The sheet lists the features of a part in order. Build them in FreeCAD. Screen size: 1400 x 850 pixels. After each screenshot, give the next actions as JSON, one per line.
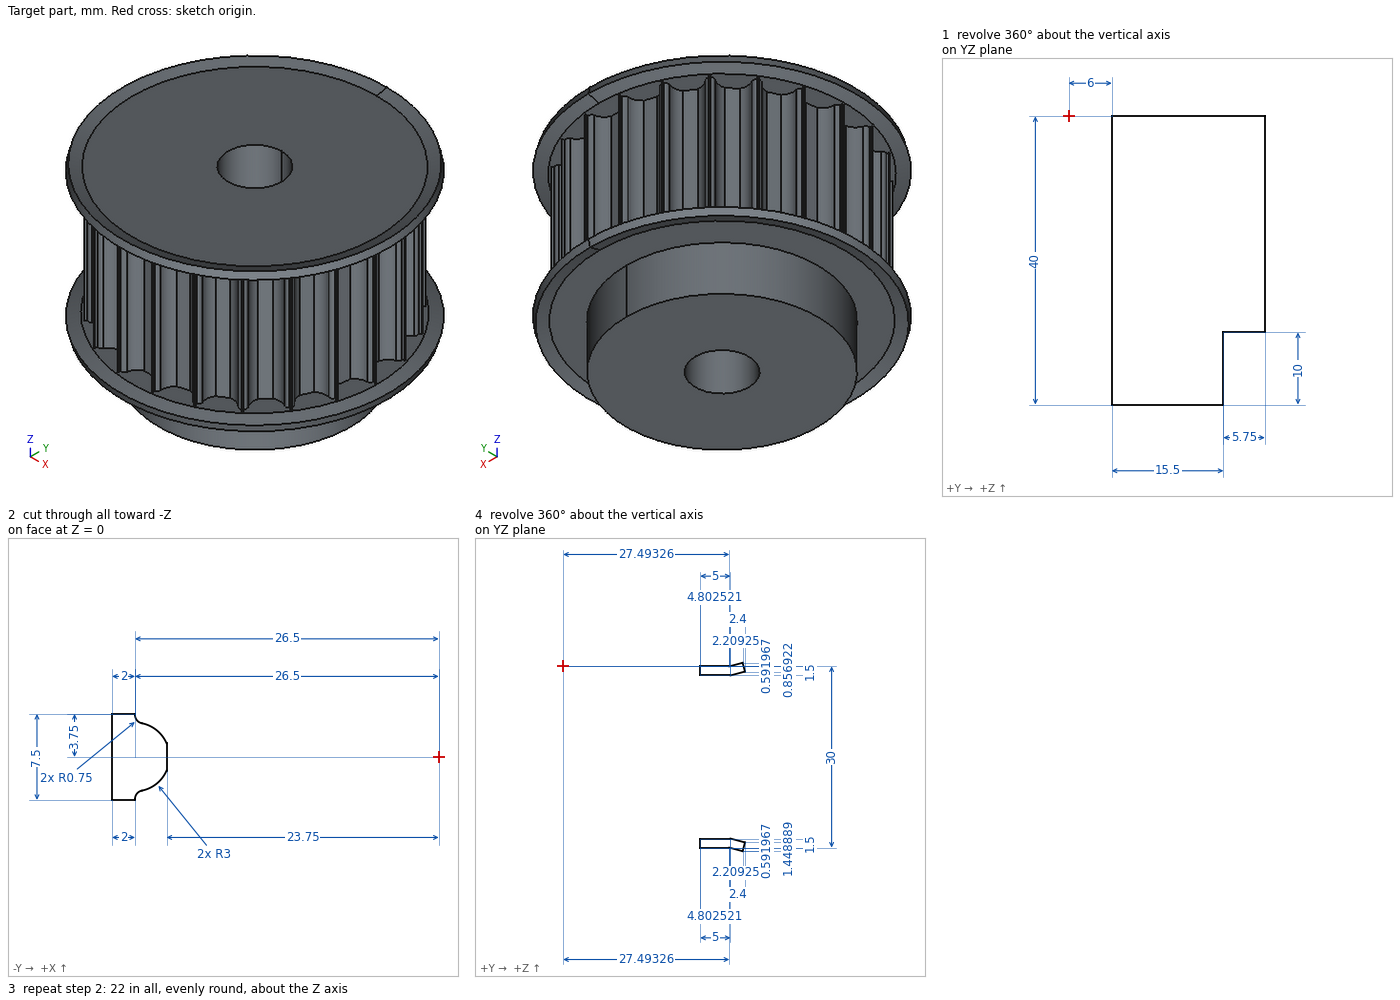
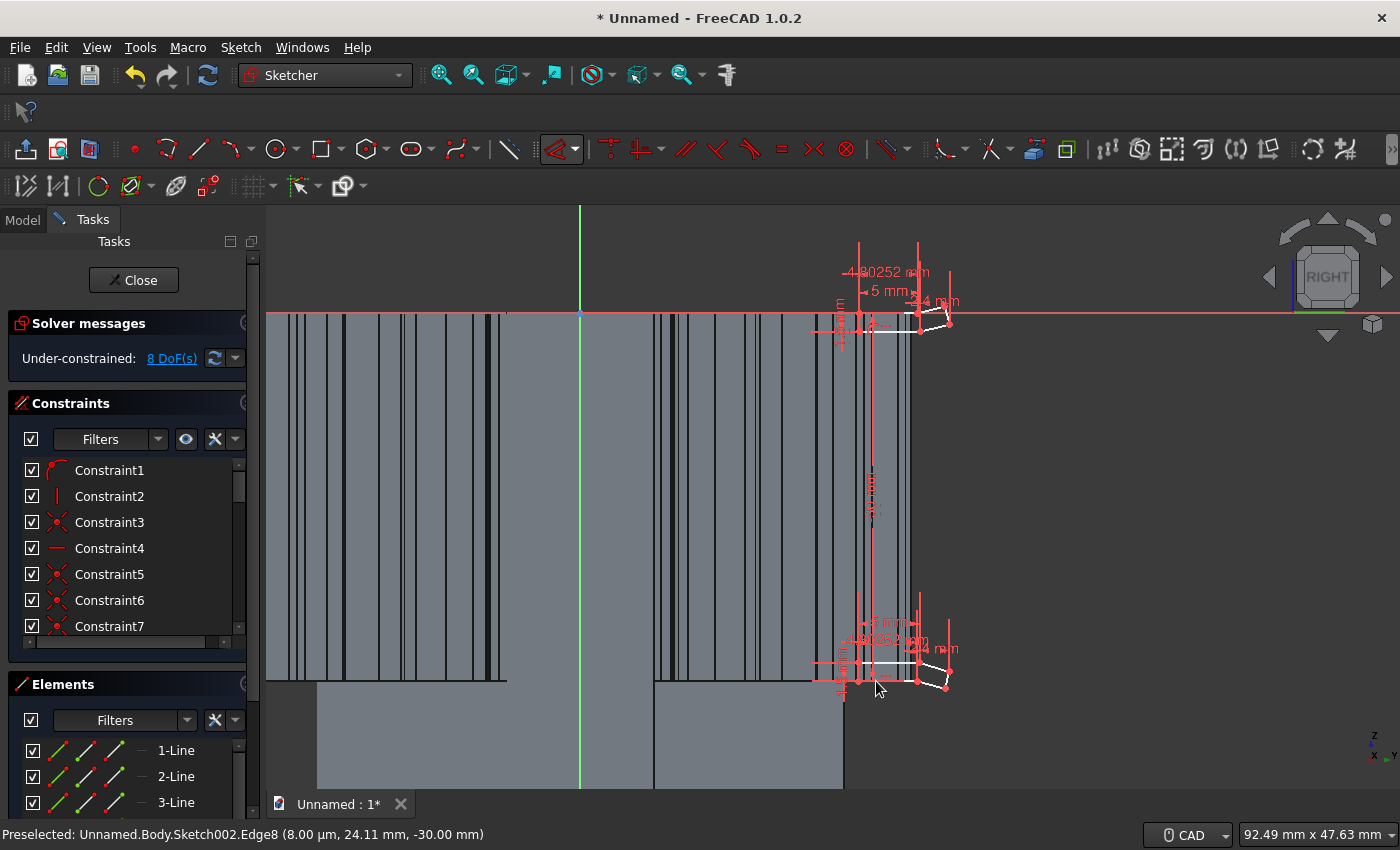
{"action": "scroll", "coordinate": [929, 311], "scroll_direction": "up", "scroll_amount": 2}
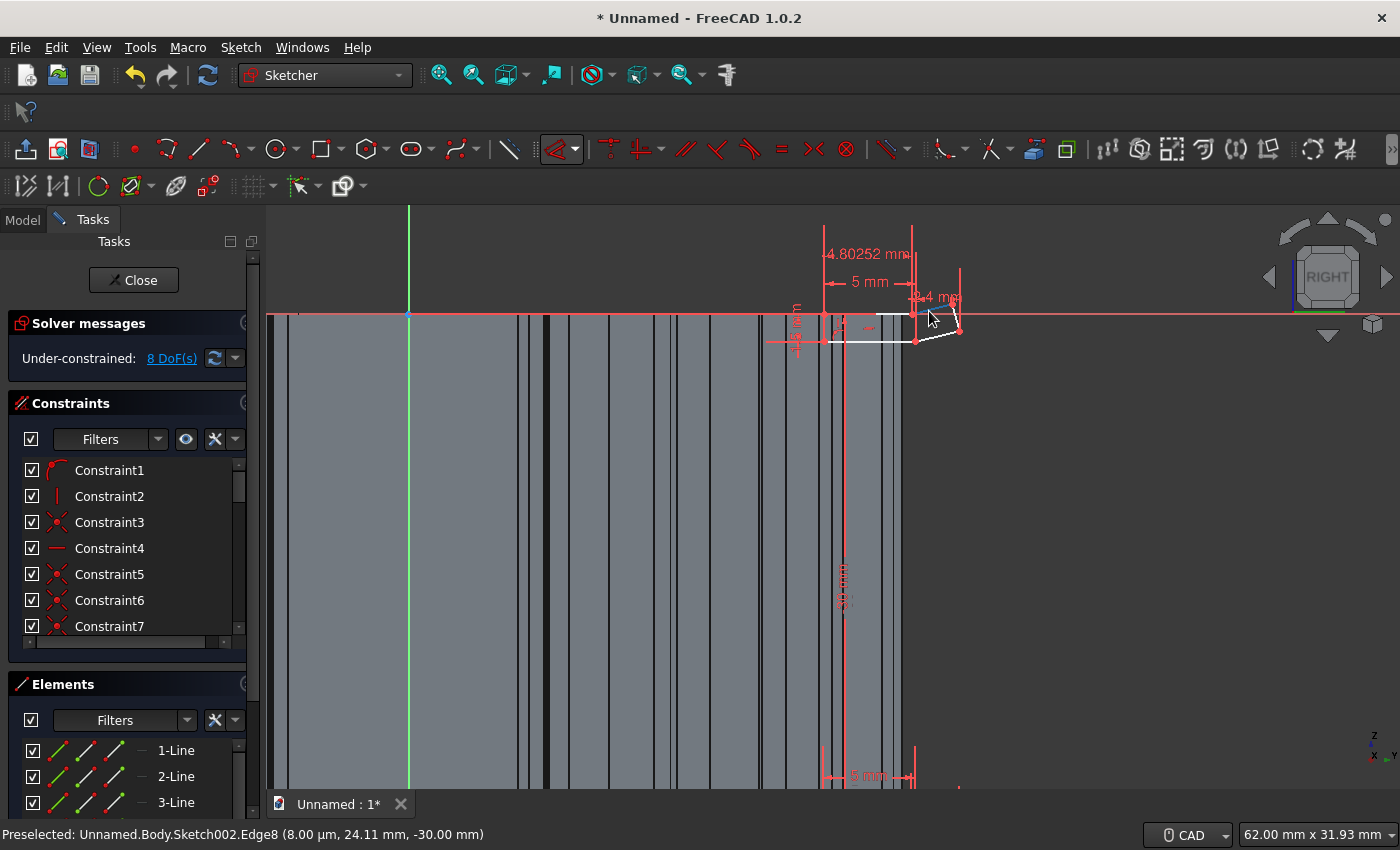
{"action": "left_click", "coordinate": [928, 310]}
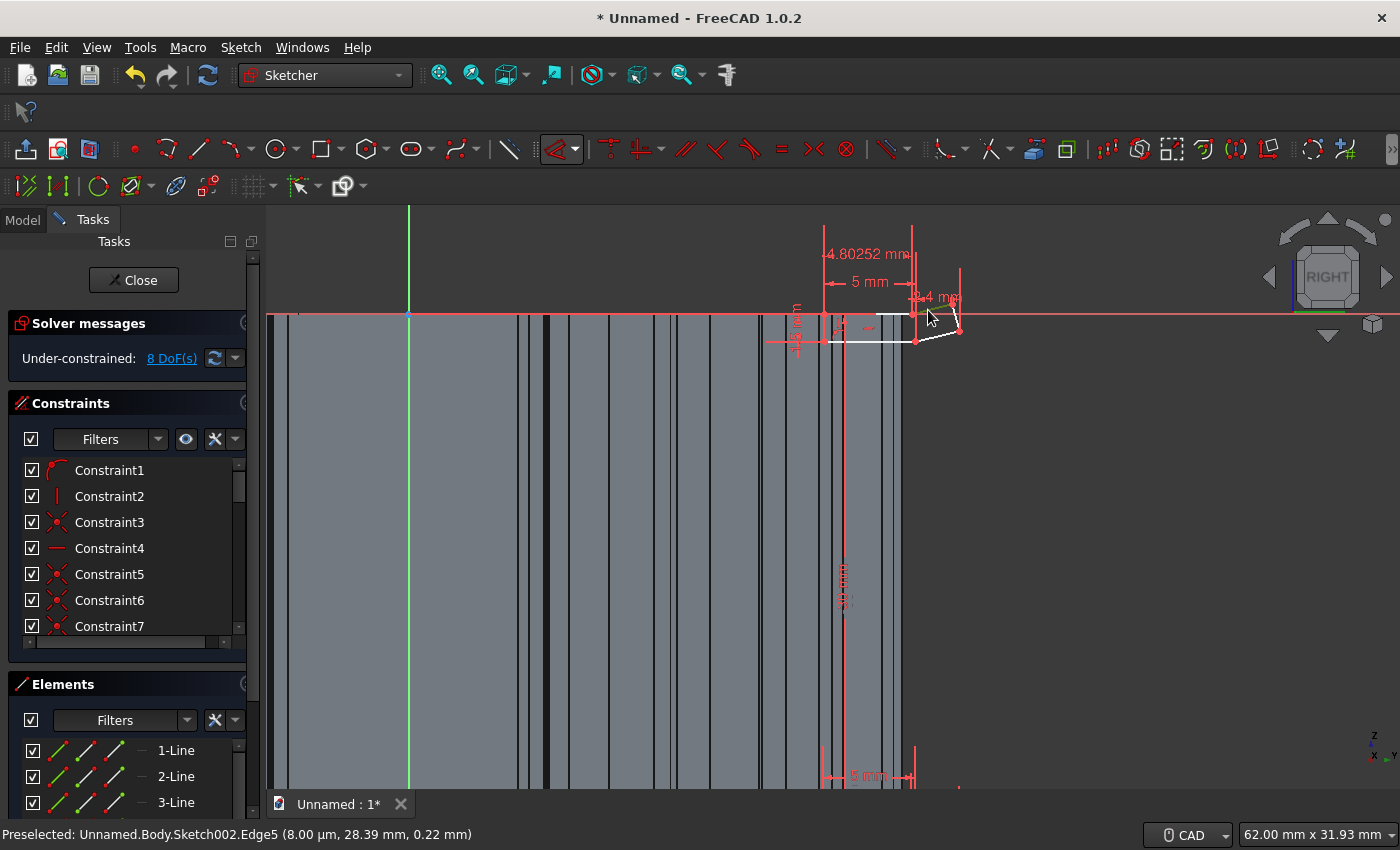
{"action": "key", "text": "l"}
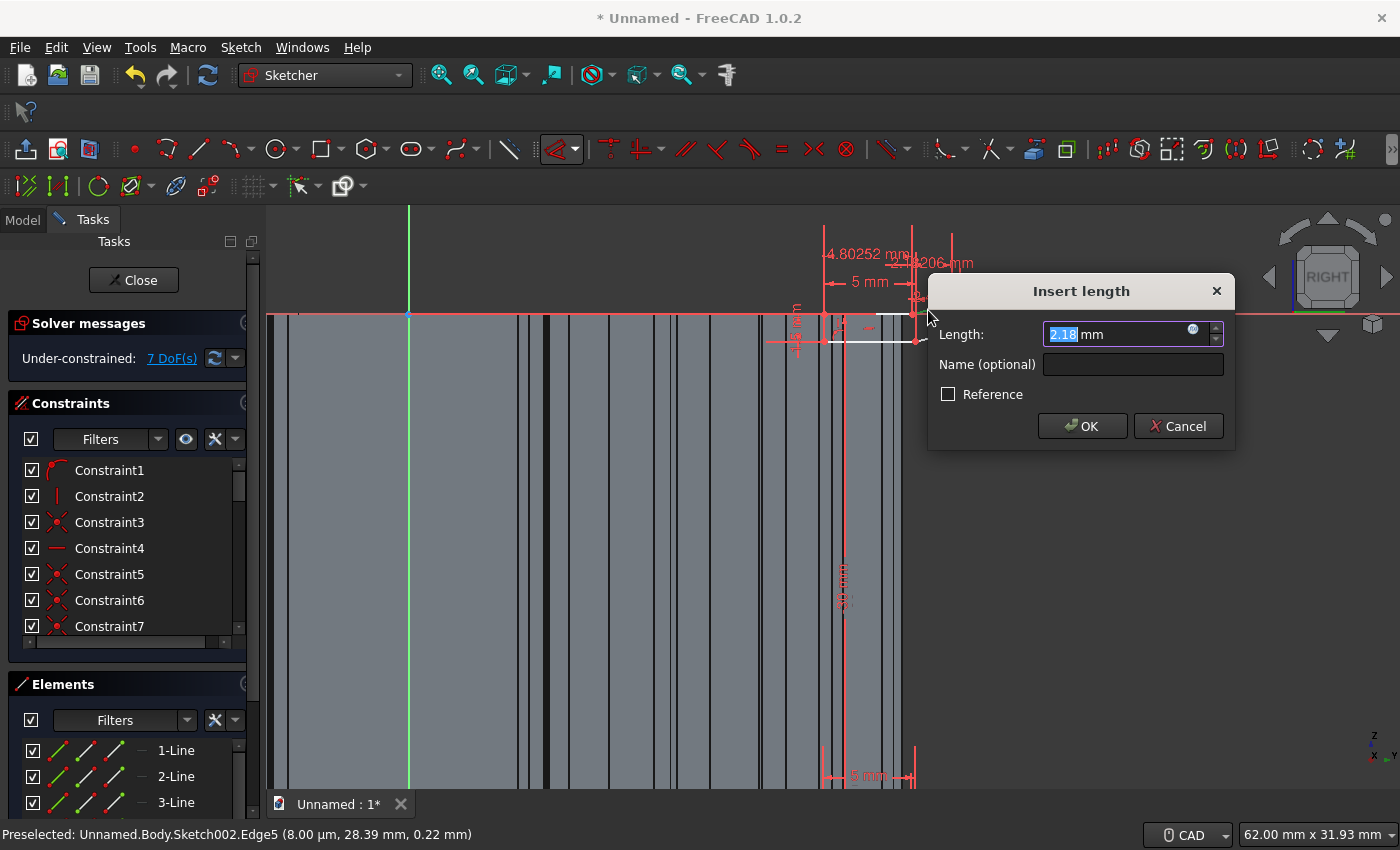
{"action": "type", "text": "2.20925"}
{"action": "key", "text": "Return"}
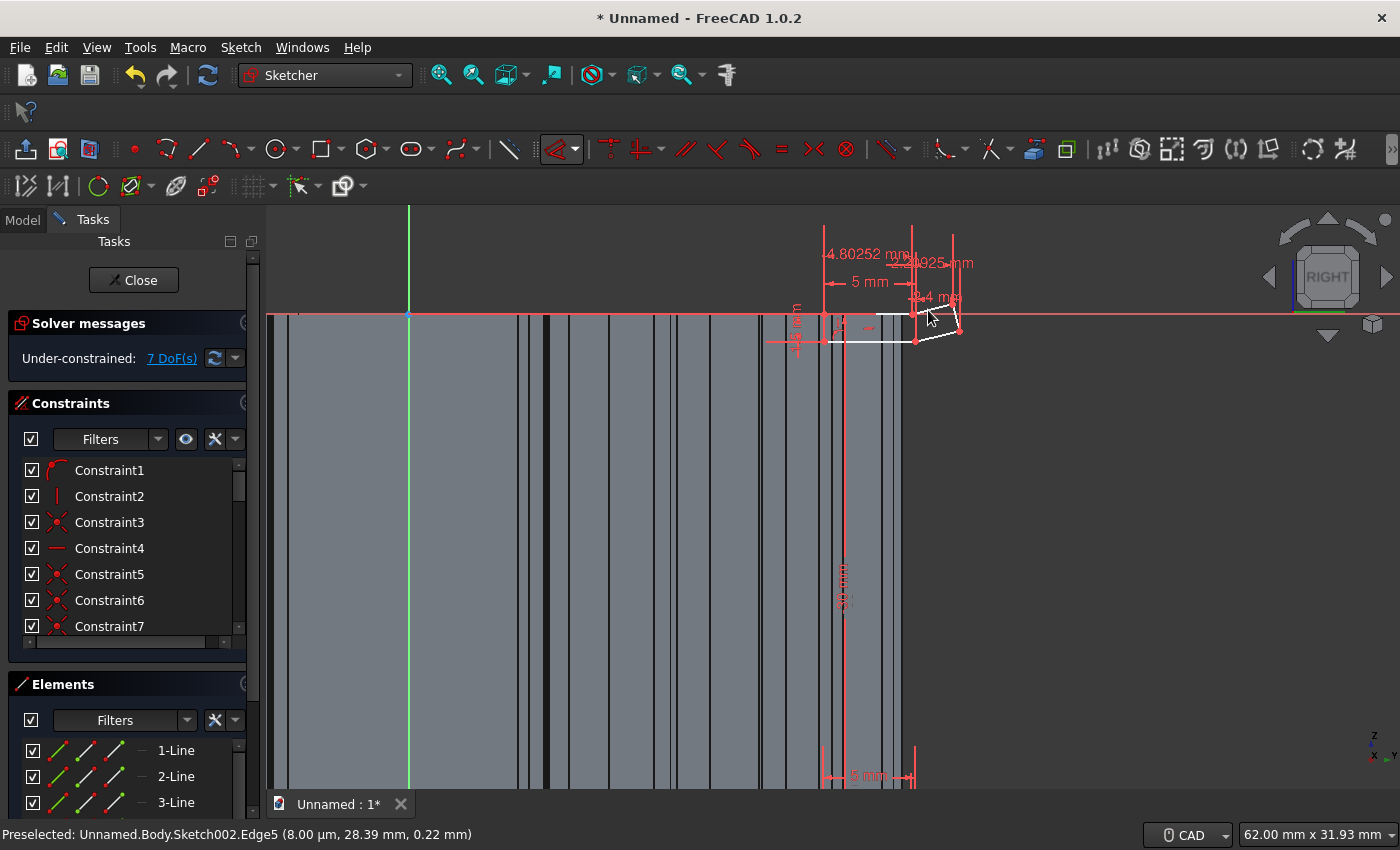
{"action": "scroll", "coordinate": [929, 310], "scroll_direction": "down", "scroll_amount": 2}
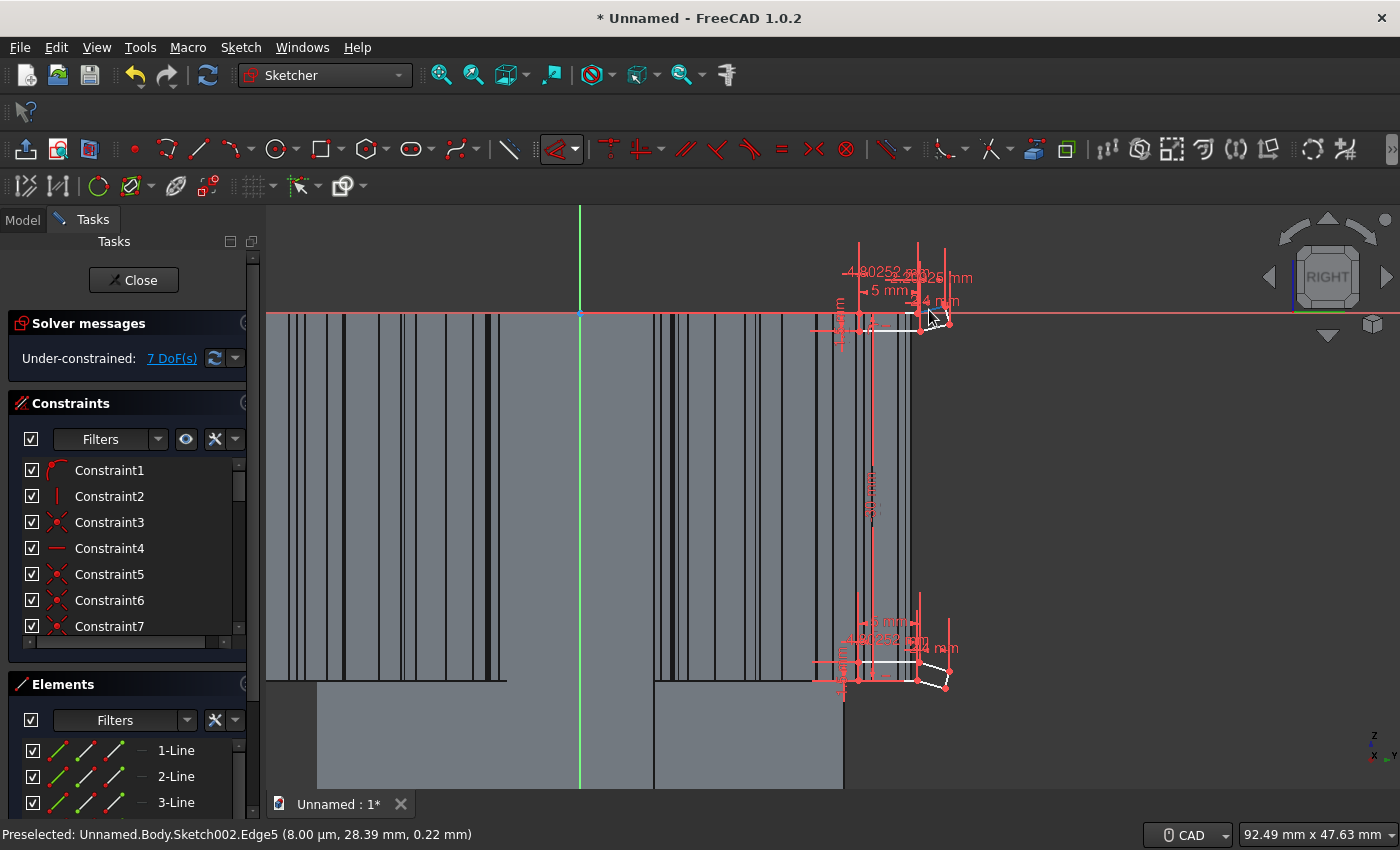
{"action": "scroll", "coordinate": [926, 683], "scroll_direction": "up", "scroll_amount": 3}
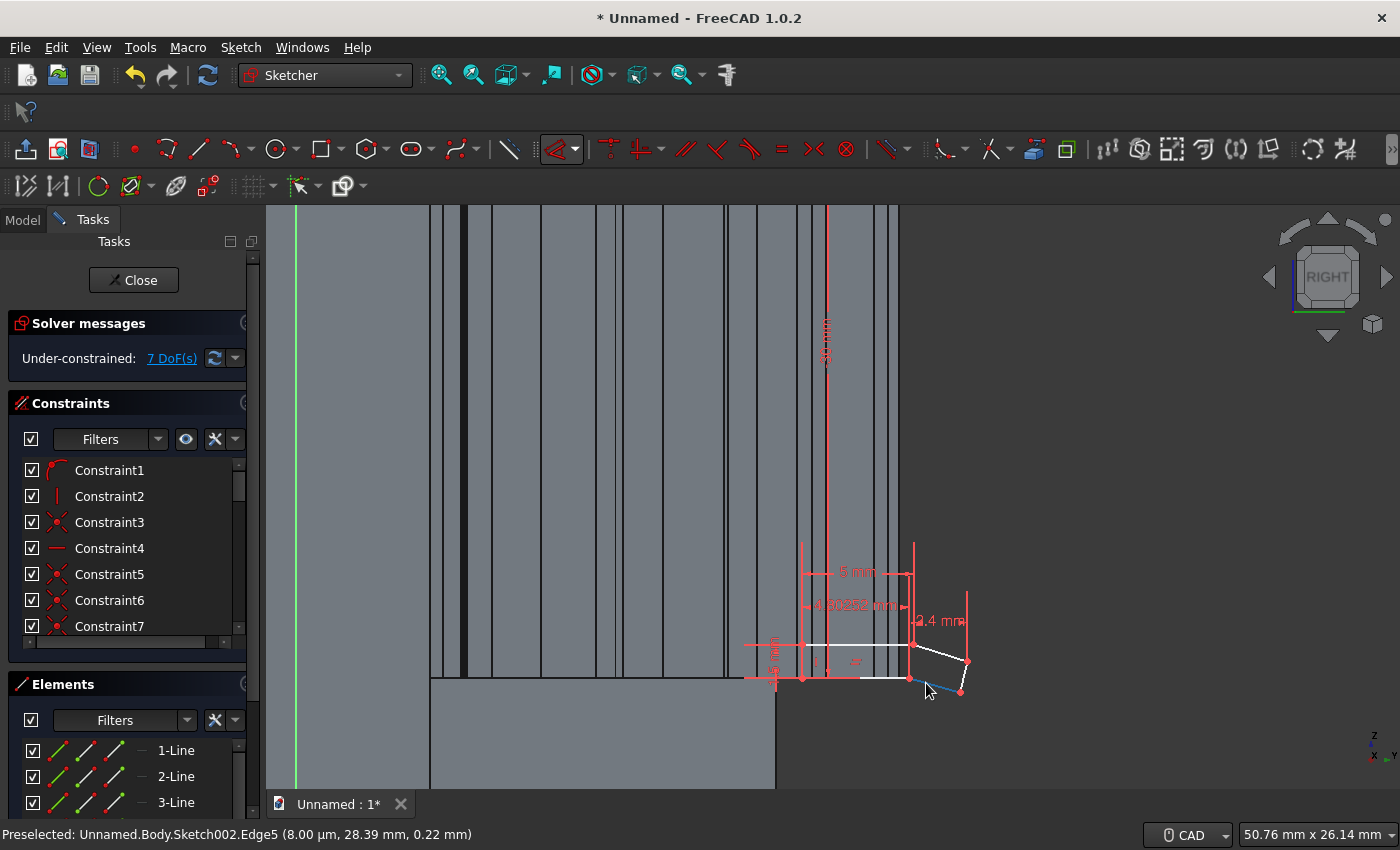
{"action": "left_click", "coordinate": [925, 683]}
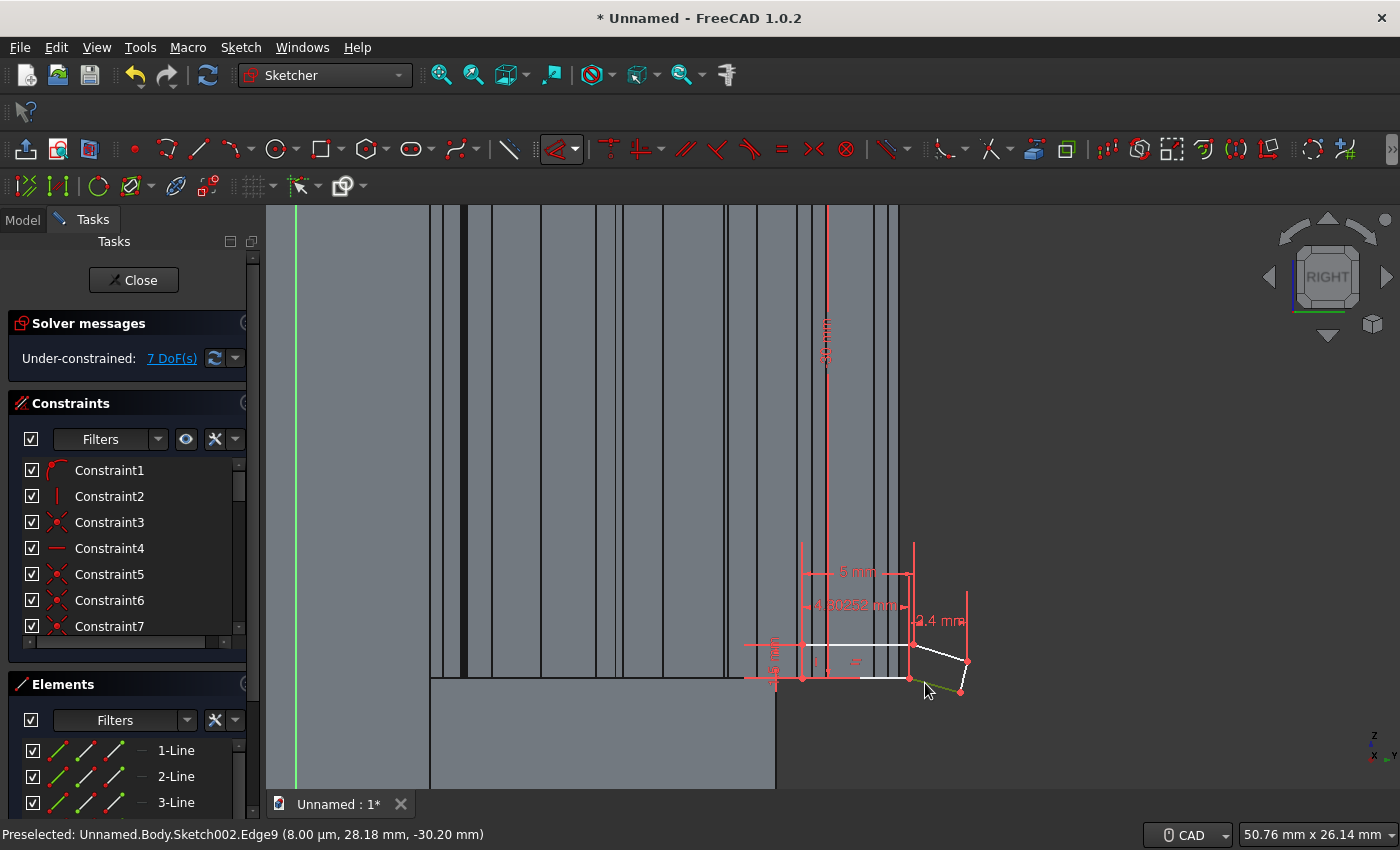
{"action": "left_click", "coordinate": [578, 150]}